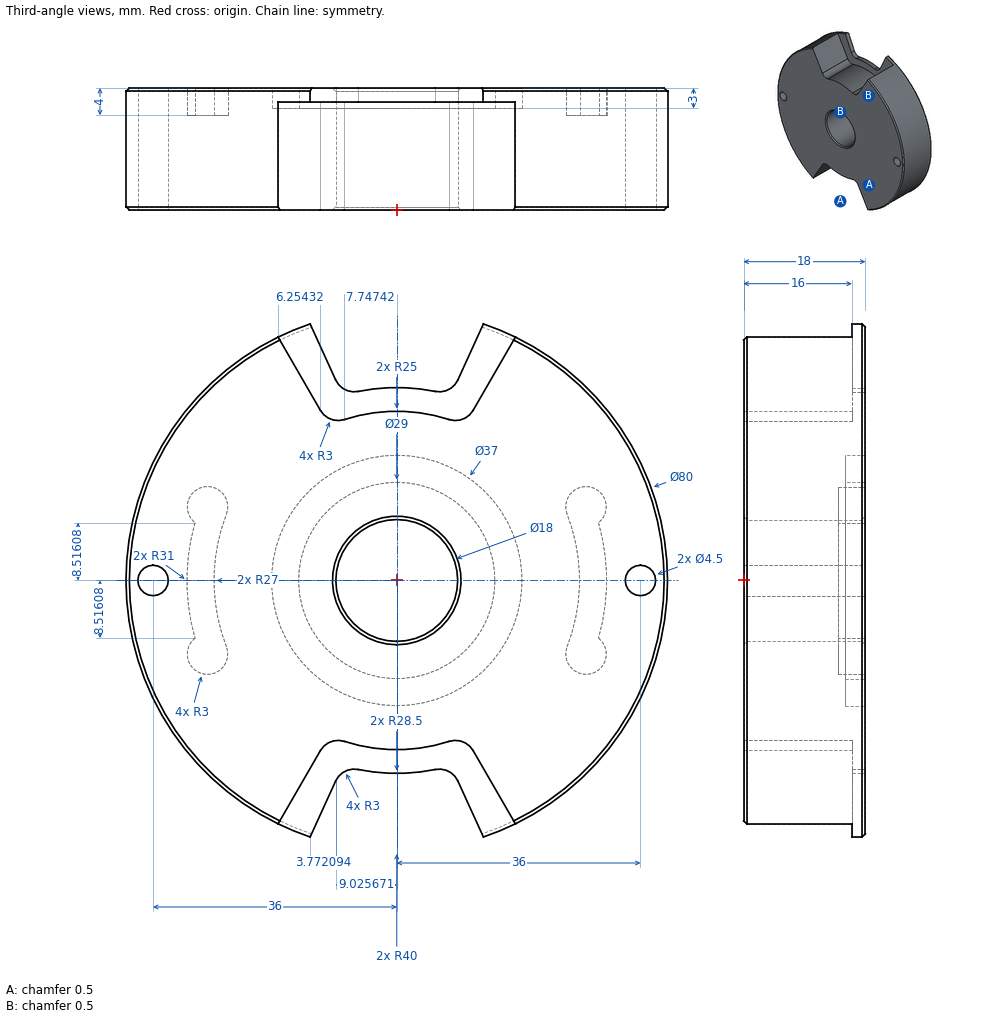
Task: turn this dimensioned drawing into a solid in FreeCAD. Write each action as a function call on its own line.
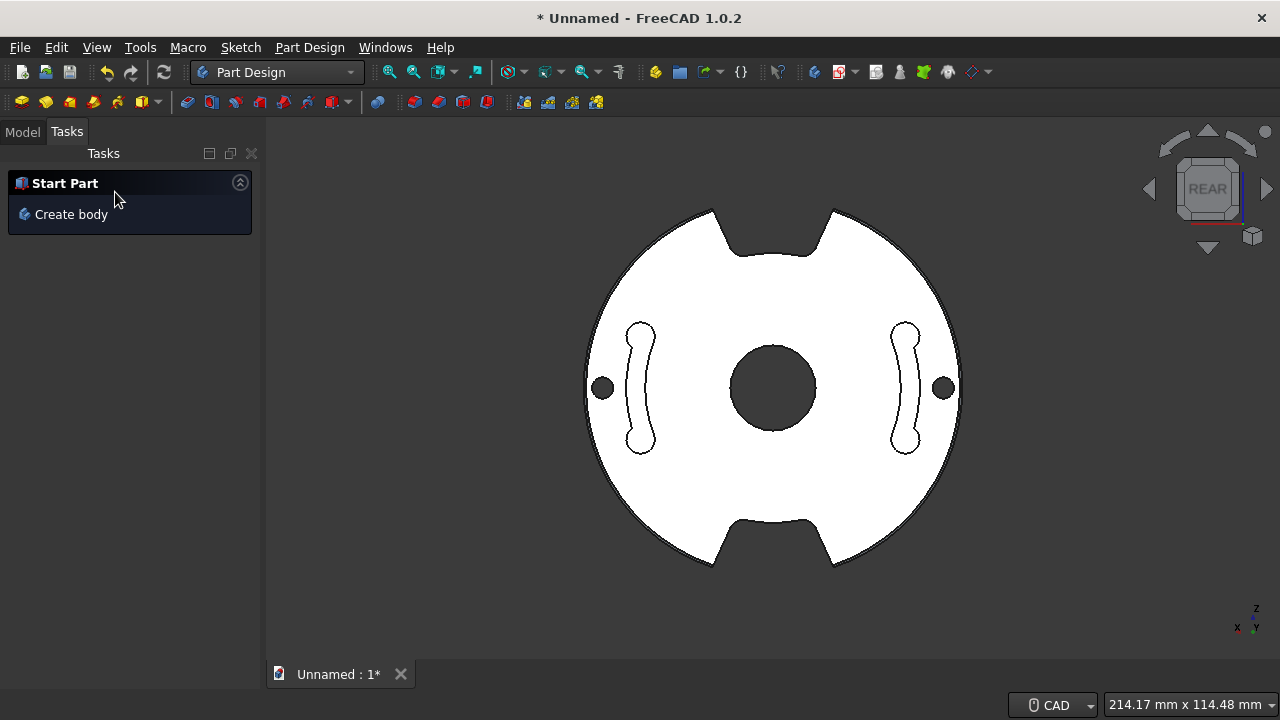
click(840, 72)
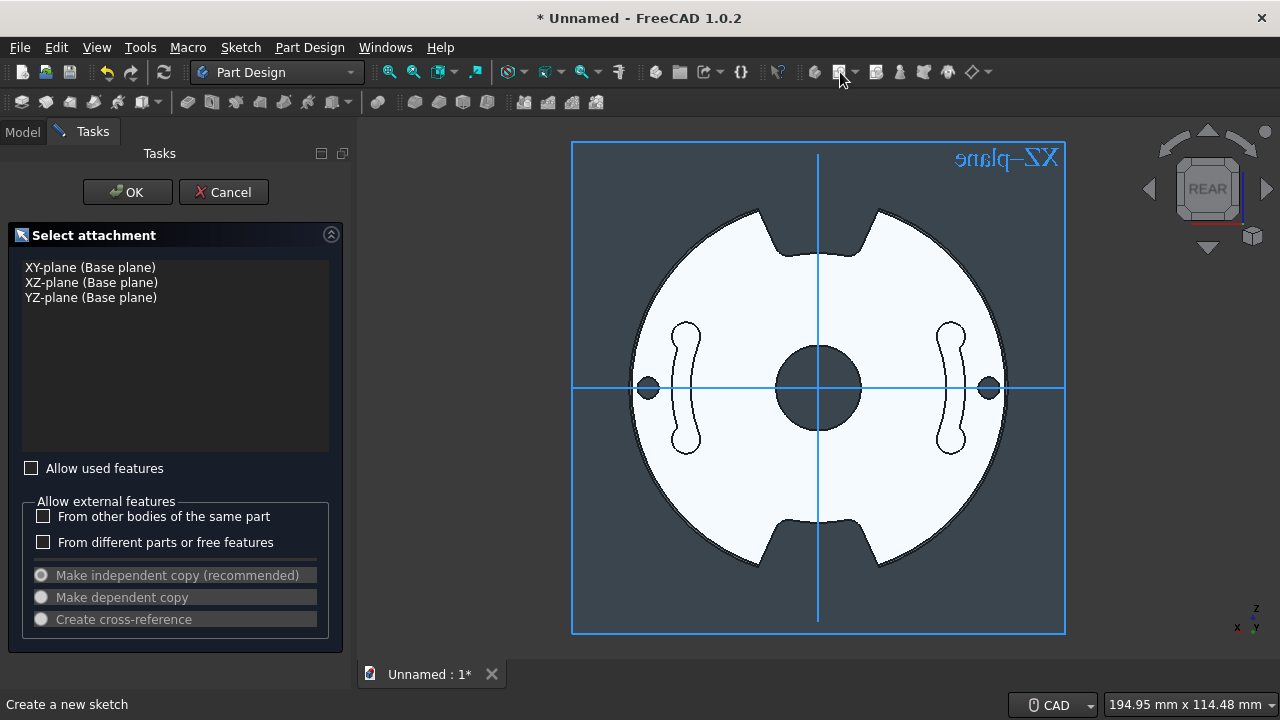
click(82, 282)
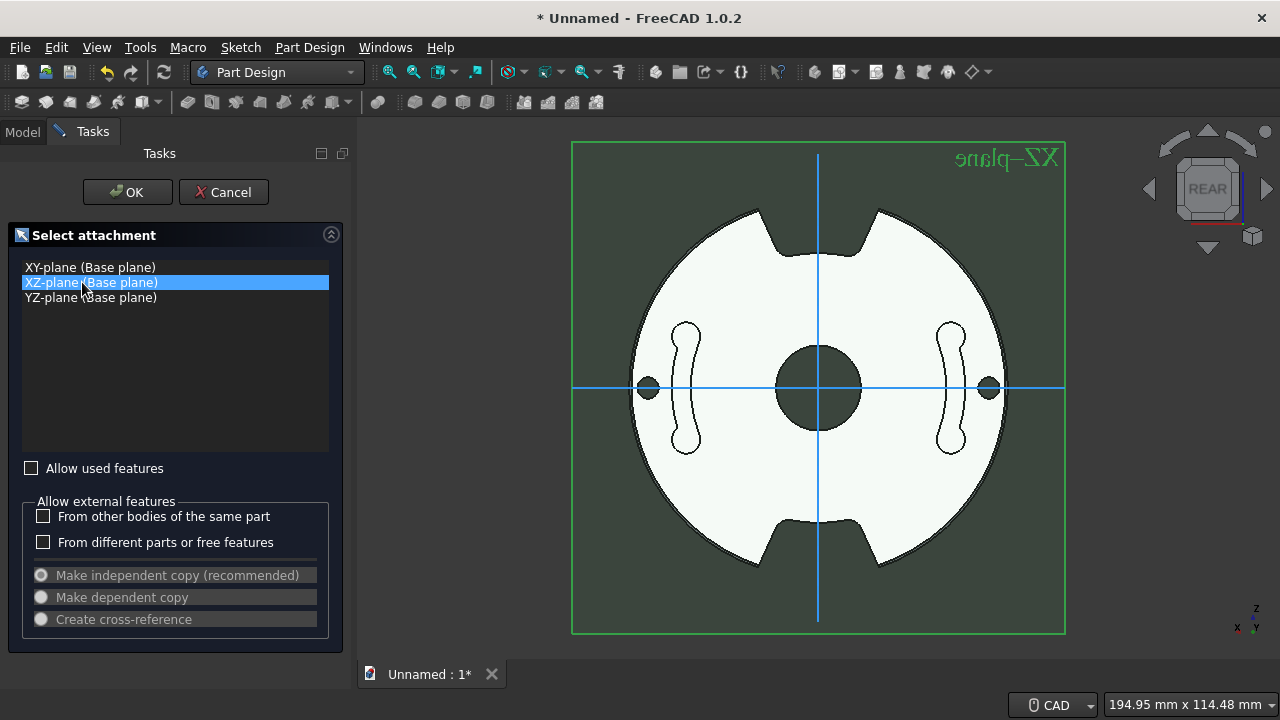
click(128, 192)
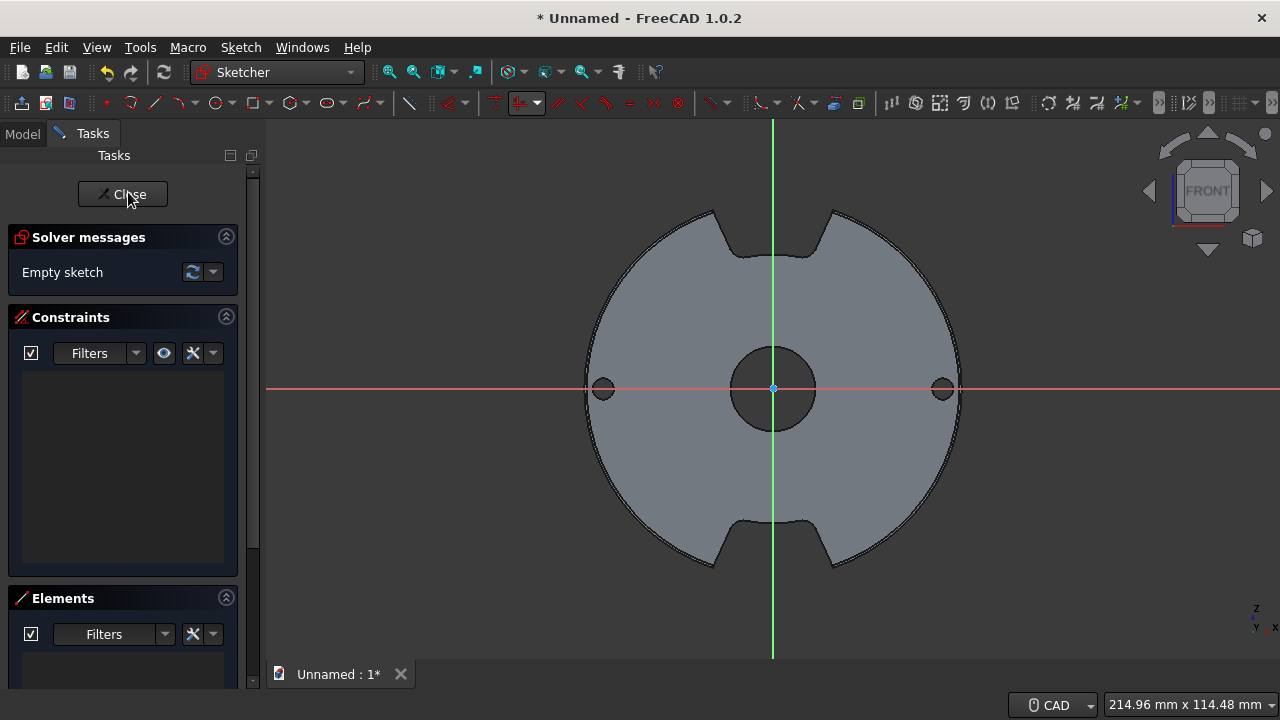
click(156, 104)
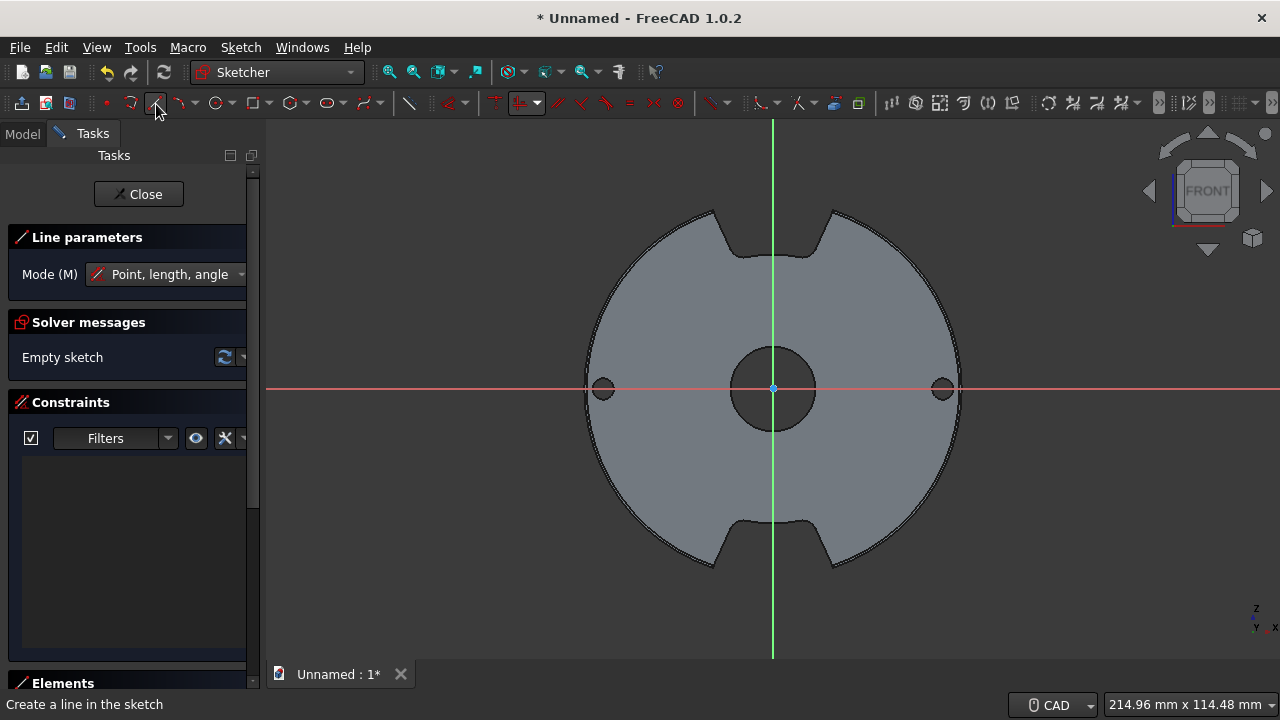
click(690, 219)
click(720, 271)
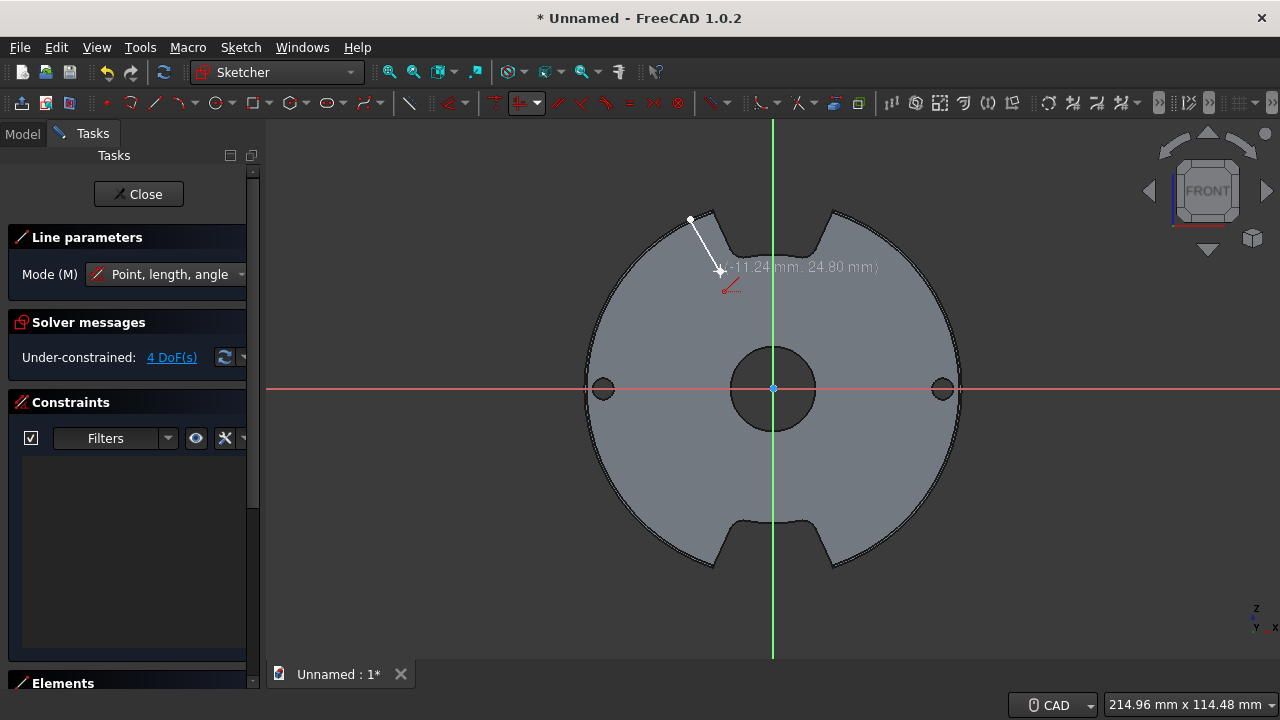
click(826, 271)
click(856, 219)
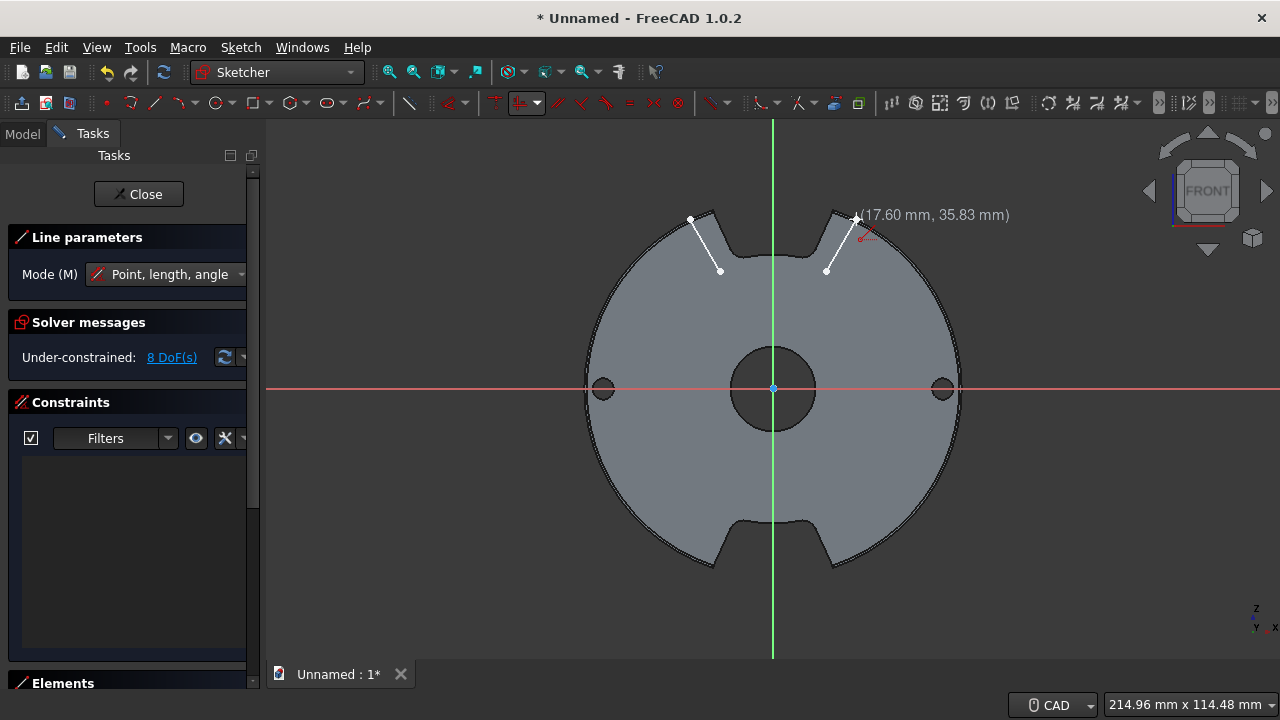
click(180, 104)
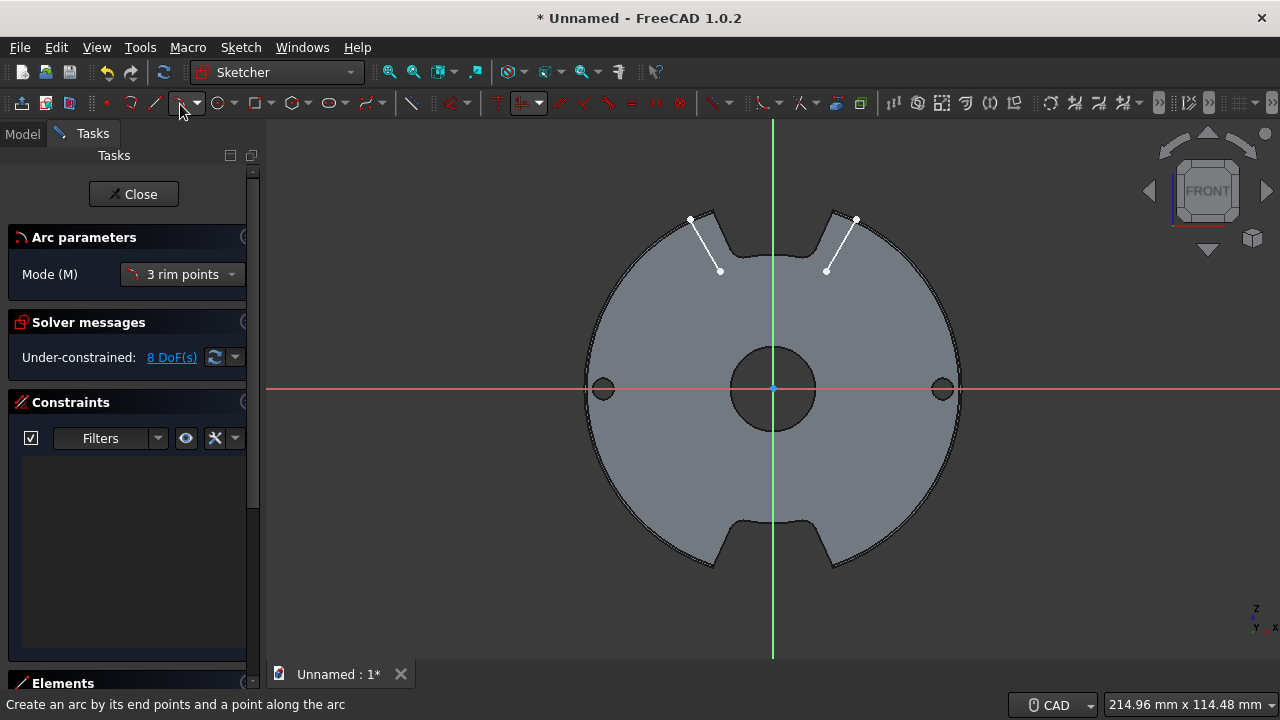
click(720, 272)
click(736, 277)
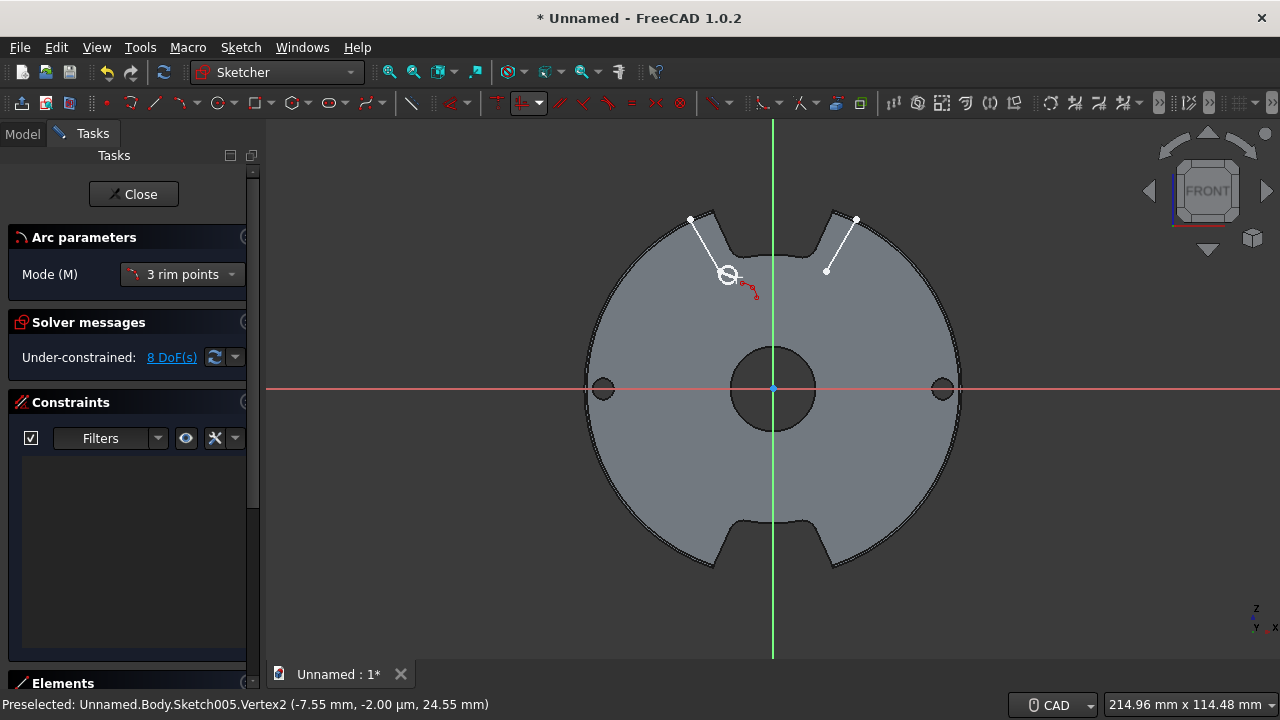
scroll(727, 277, up, 9)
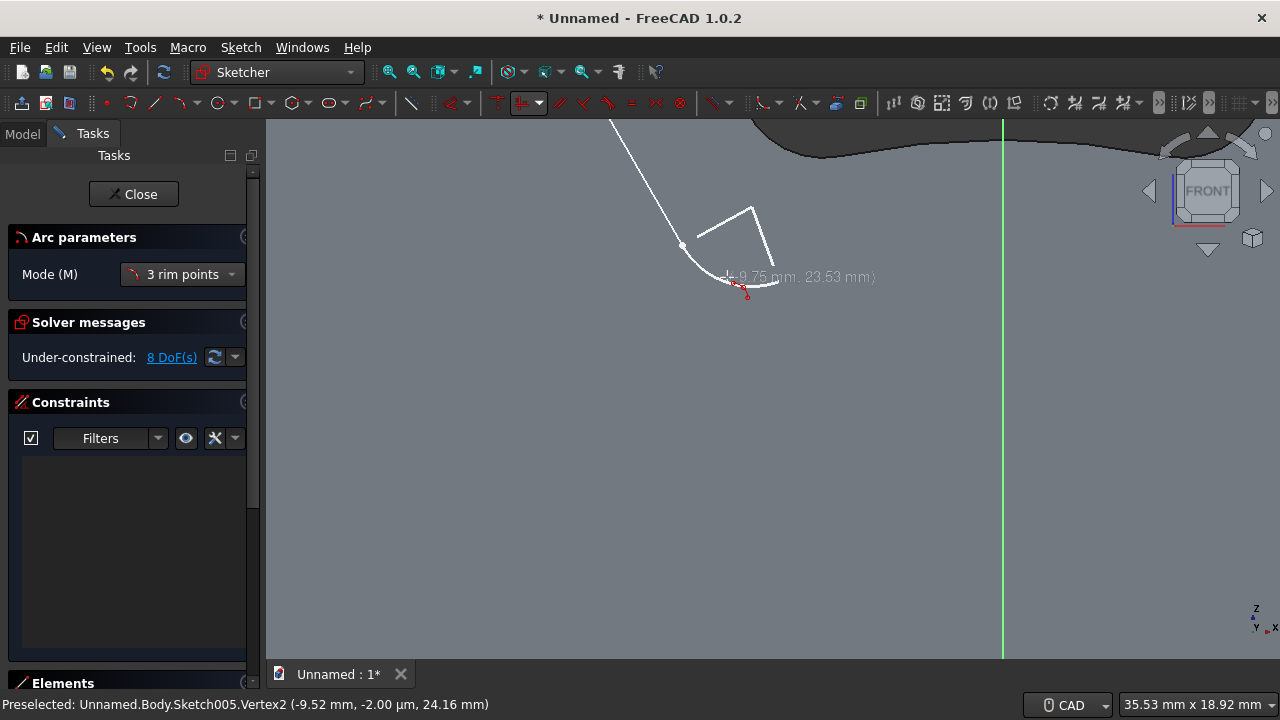
click(725, 273)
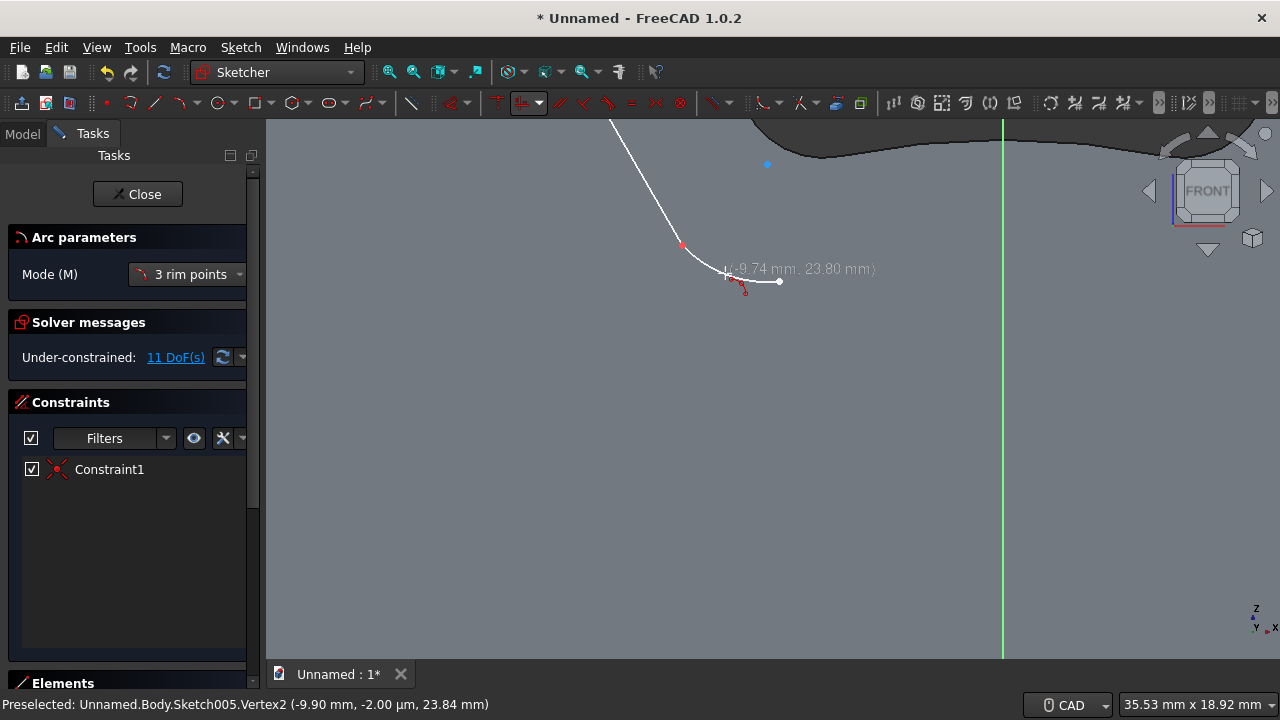
scroll(645, 277, down, 9)